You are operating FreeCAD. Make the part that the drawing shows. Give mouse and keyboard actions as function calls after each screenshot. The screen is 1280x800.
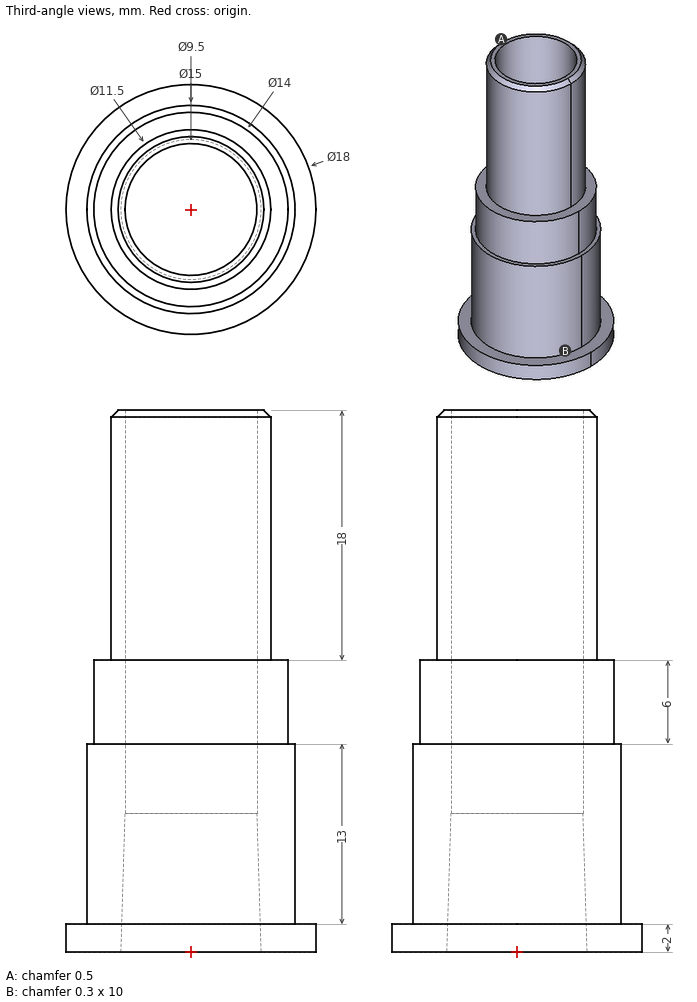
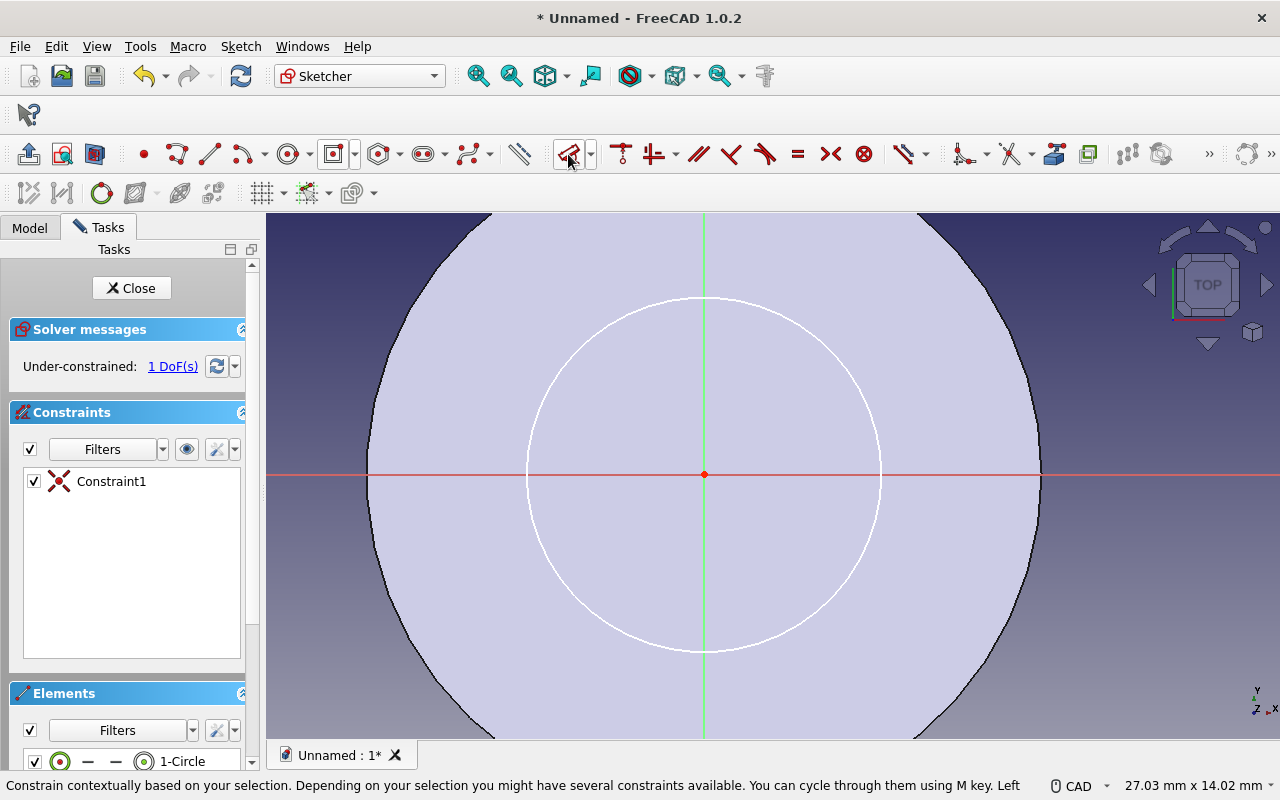
click(829, 349)
click(852, 326)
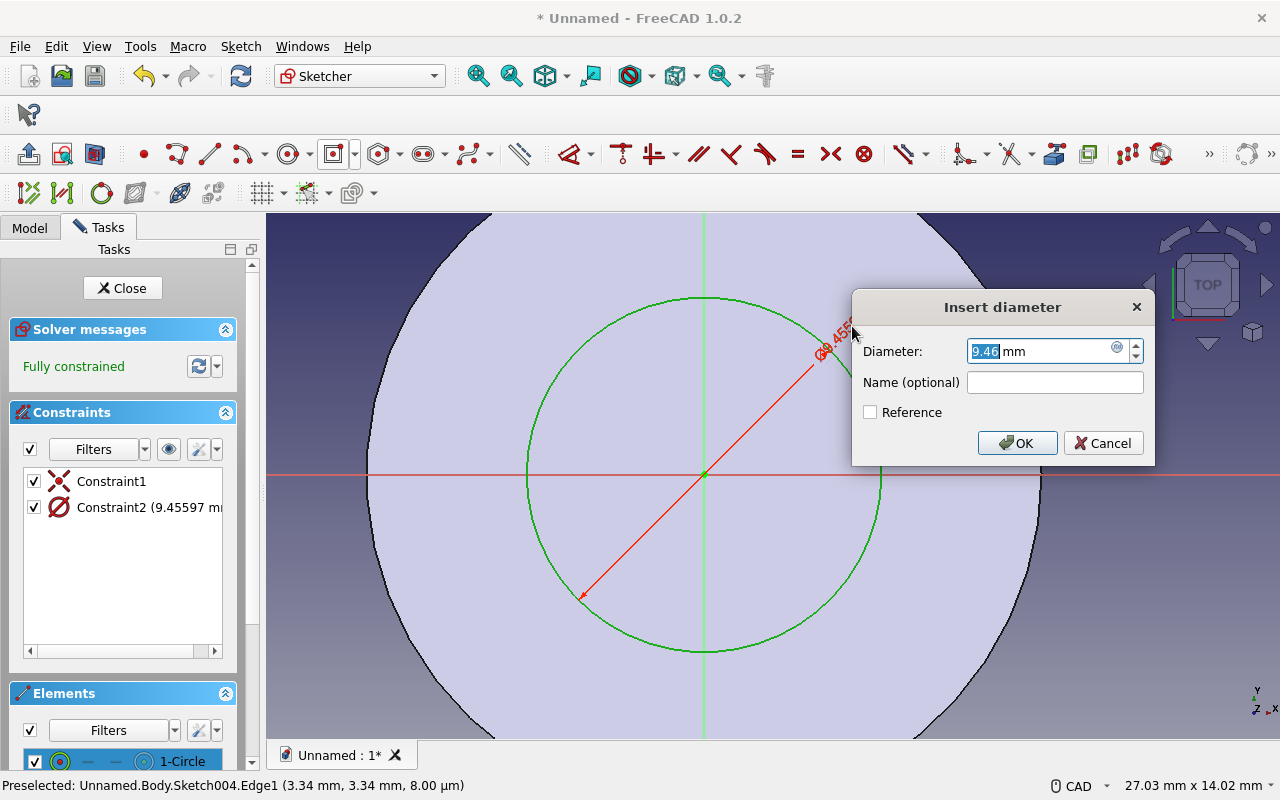
text(9.5)
key(Return)
key(Escape)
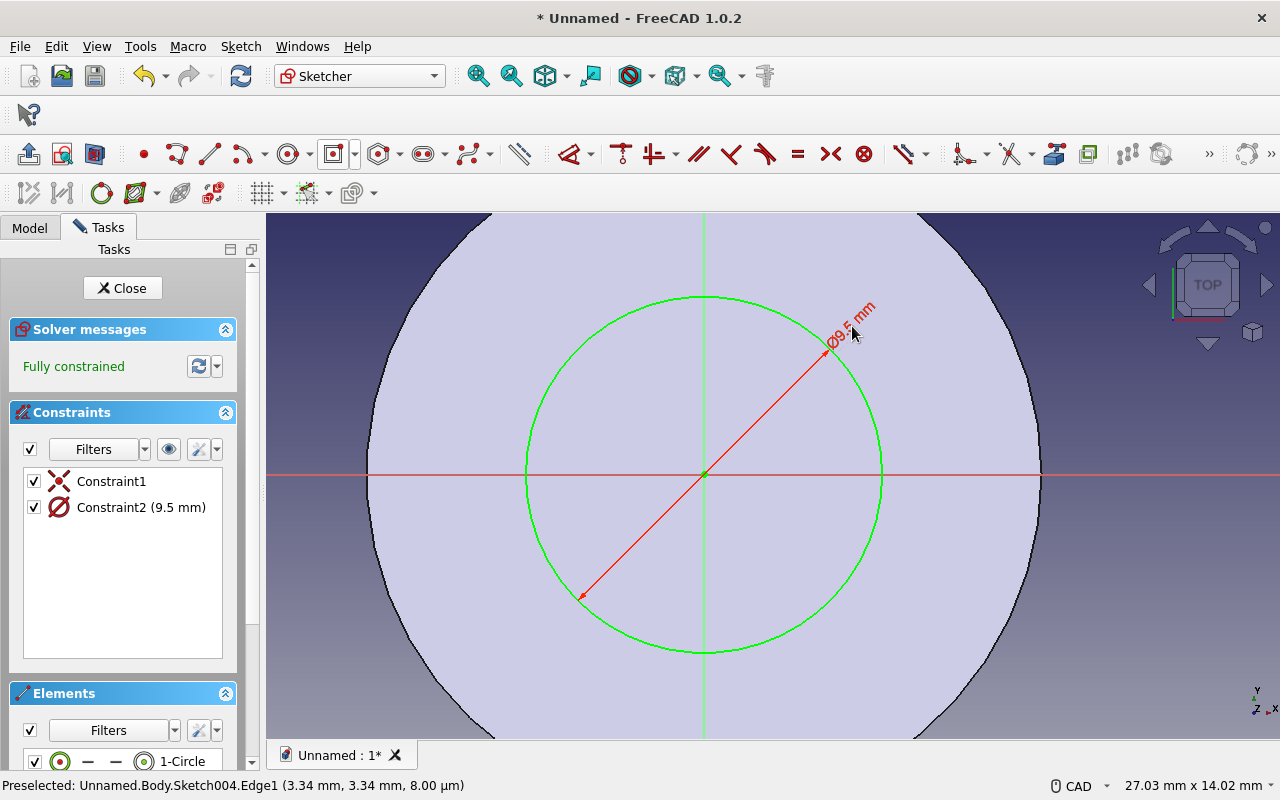
click(123, 288)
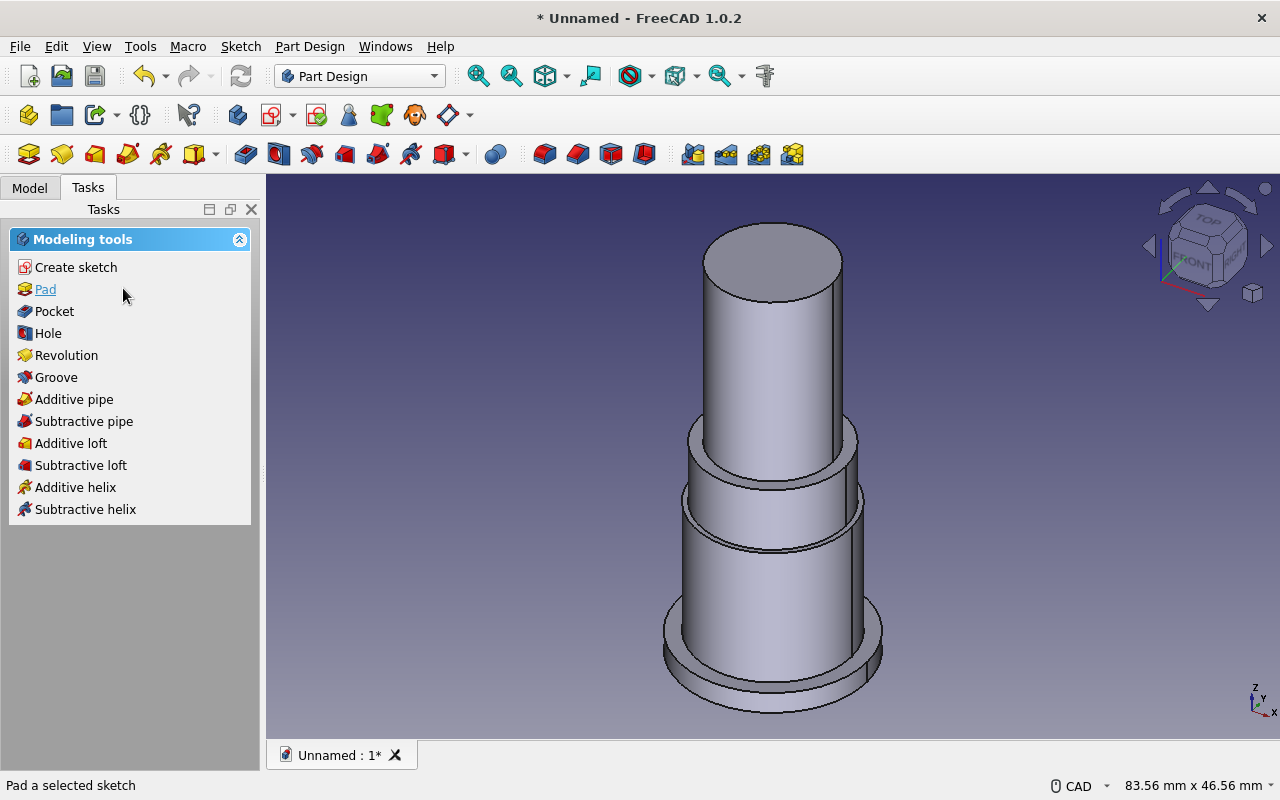
click(246, 154)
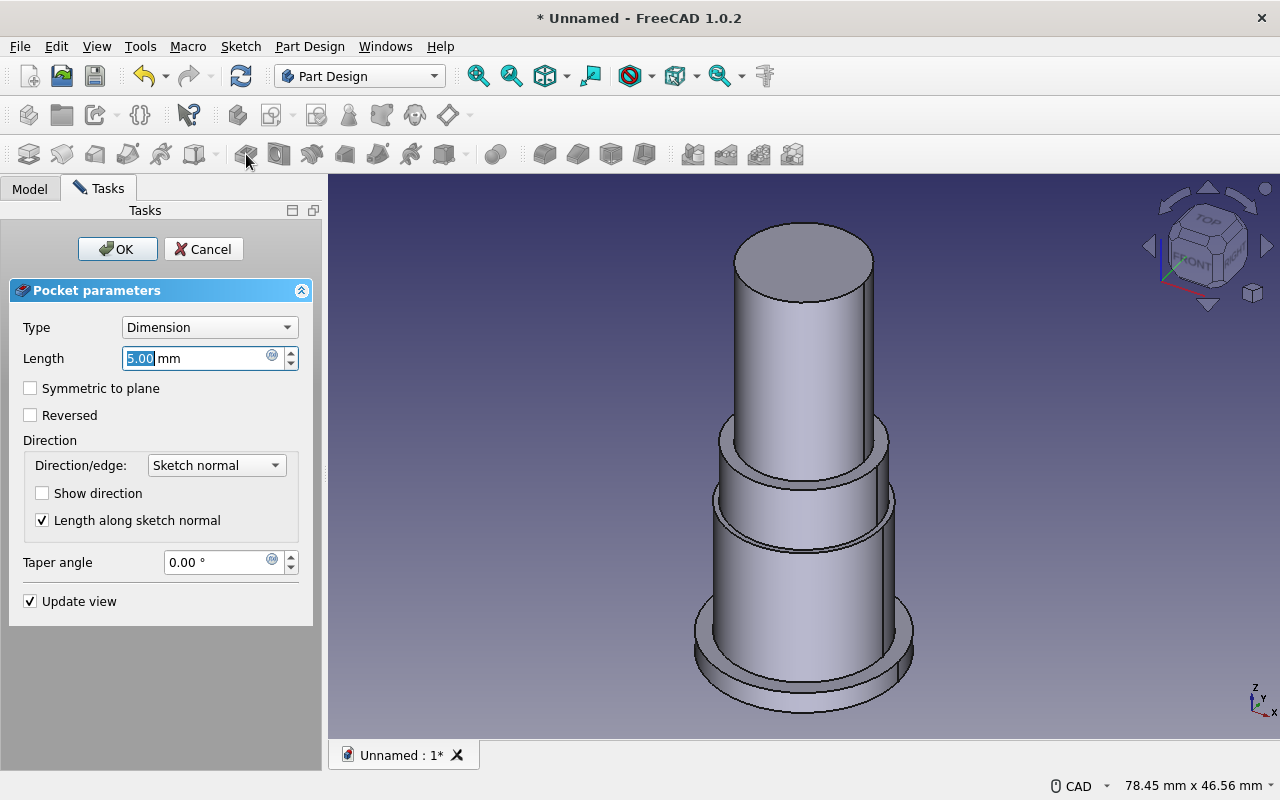
click(210, 328)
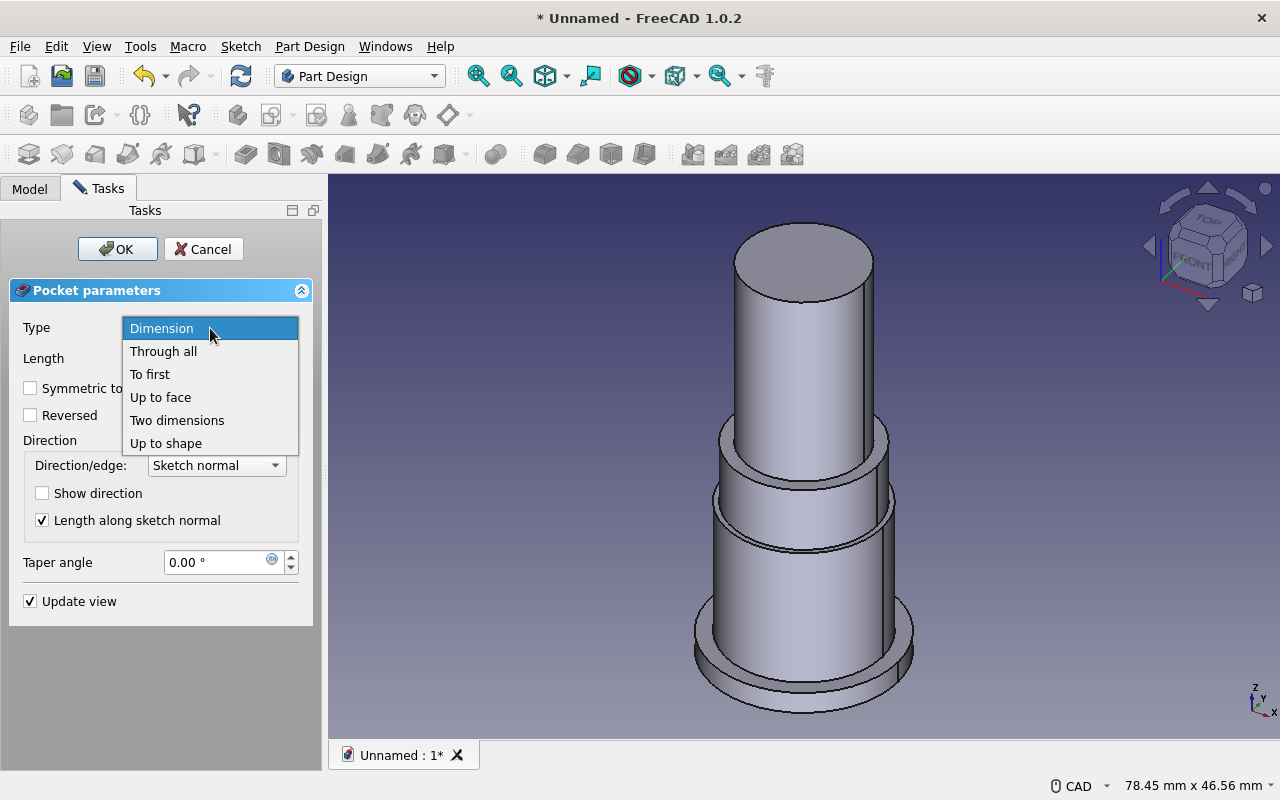
click(208, 352)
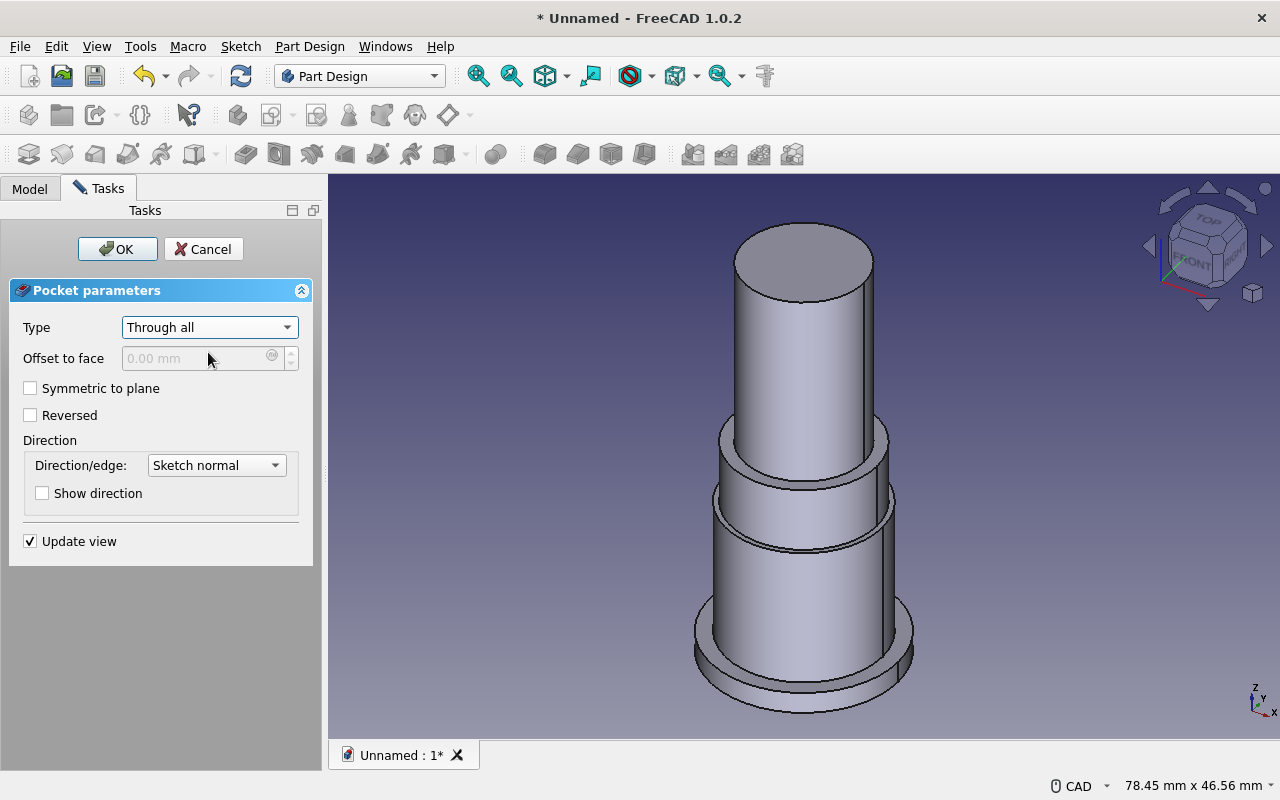
click(31, 415)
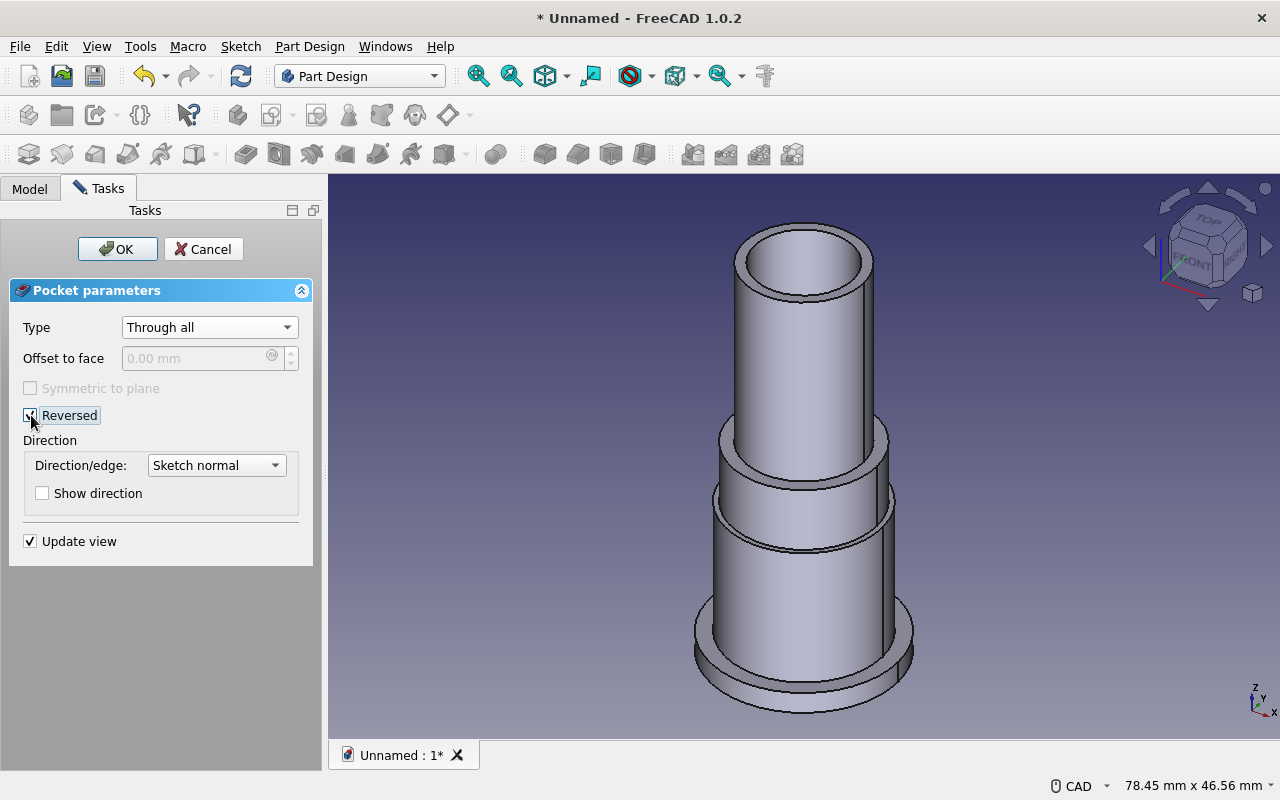
click(118, 249)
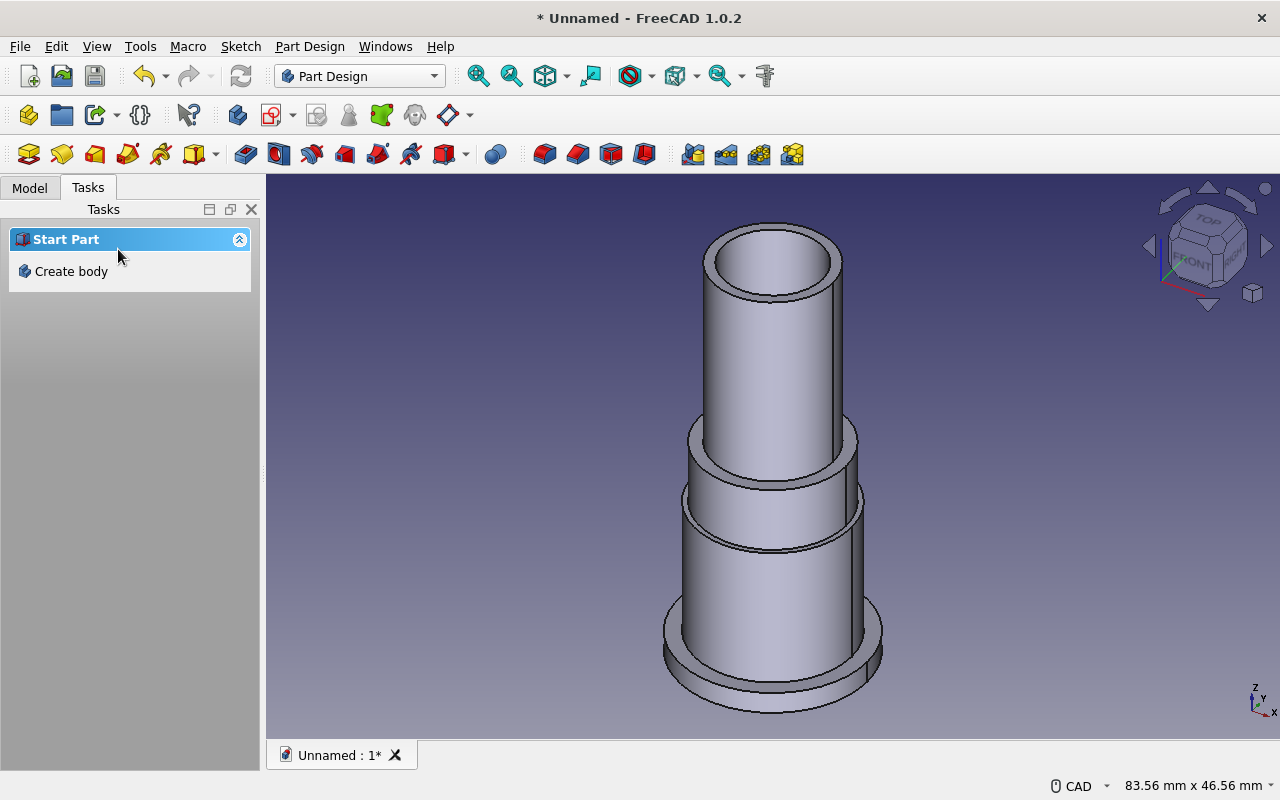
click(703, 266)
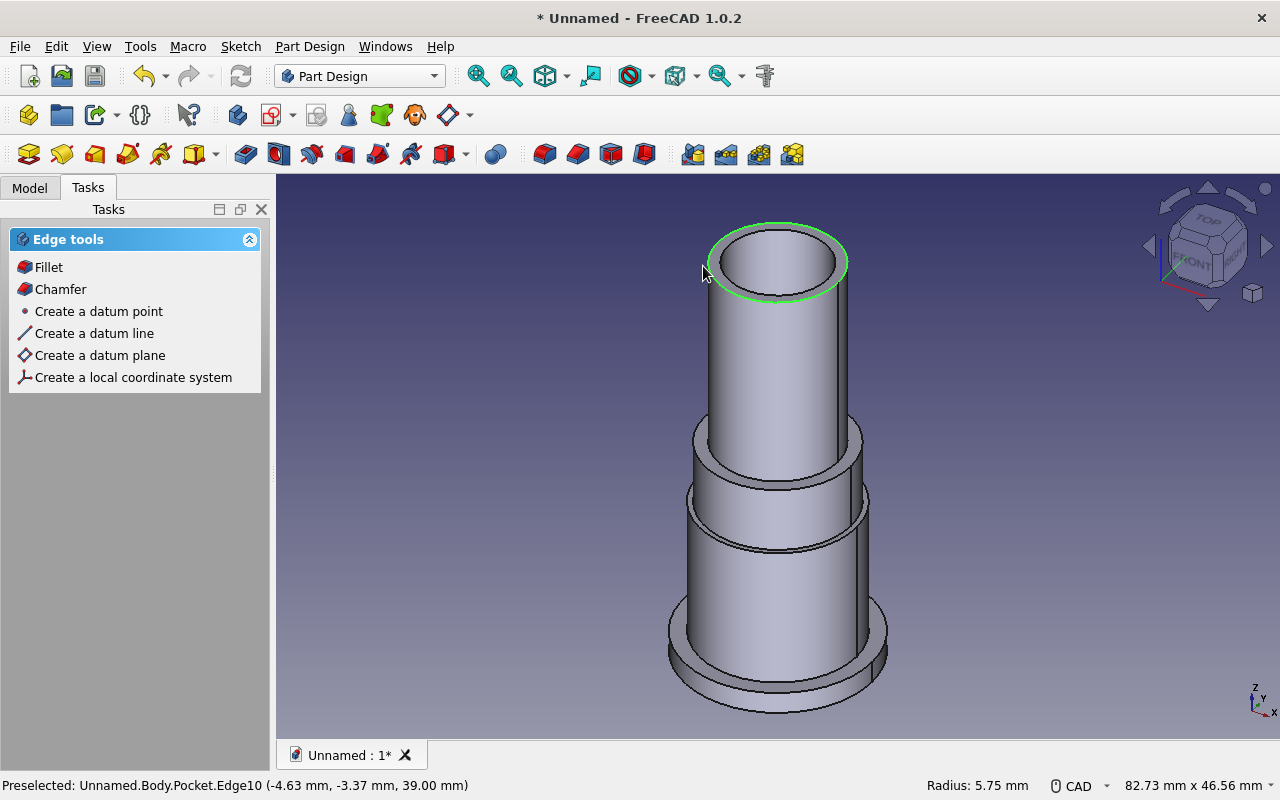
click(578, 154)